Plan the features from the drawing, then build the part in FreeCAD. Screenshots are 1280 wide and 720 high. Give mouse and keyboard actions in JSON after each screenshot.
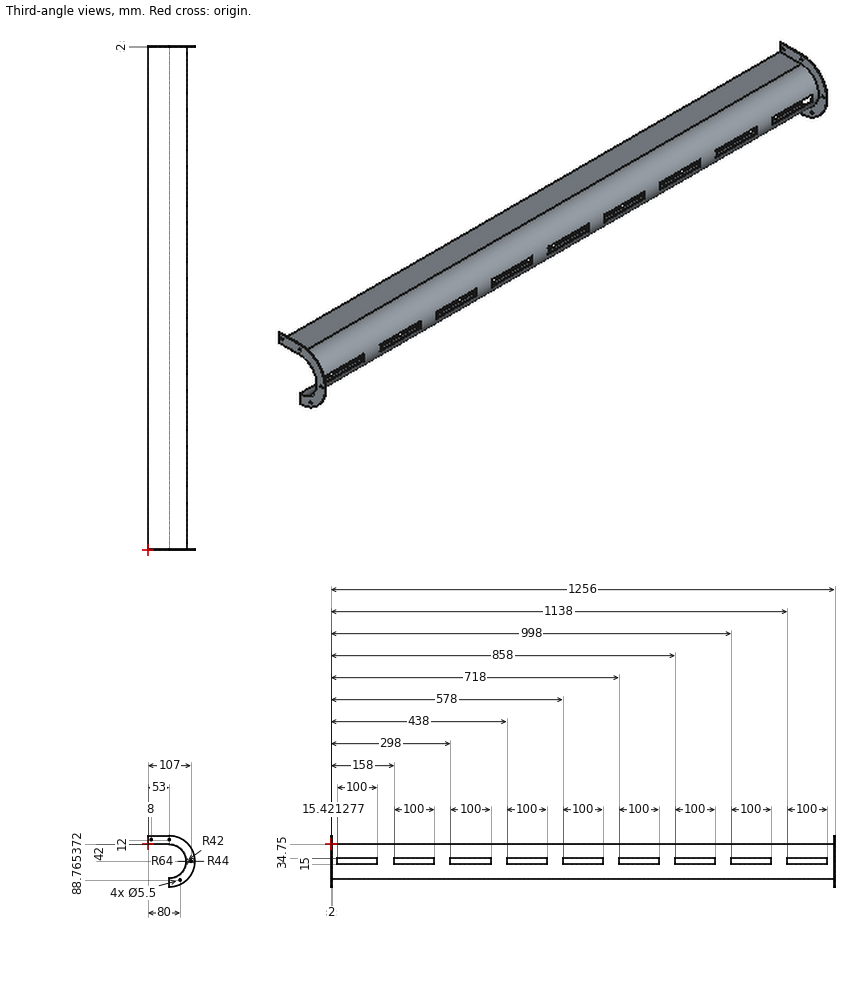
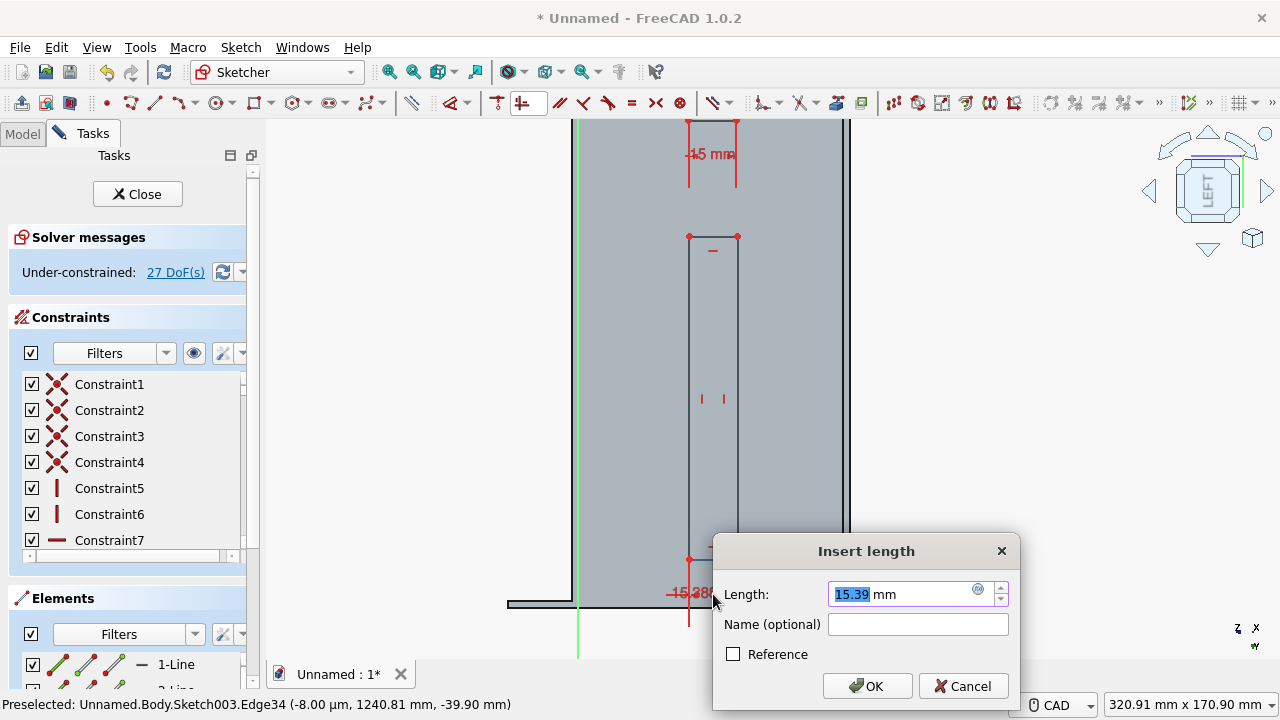
{"action": "type", "text": "15"}
{"action": "key", "text": "Return"}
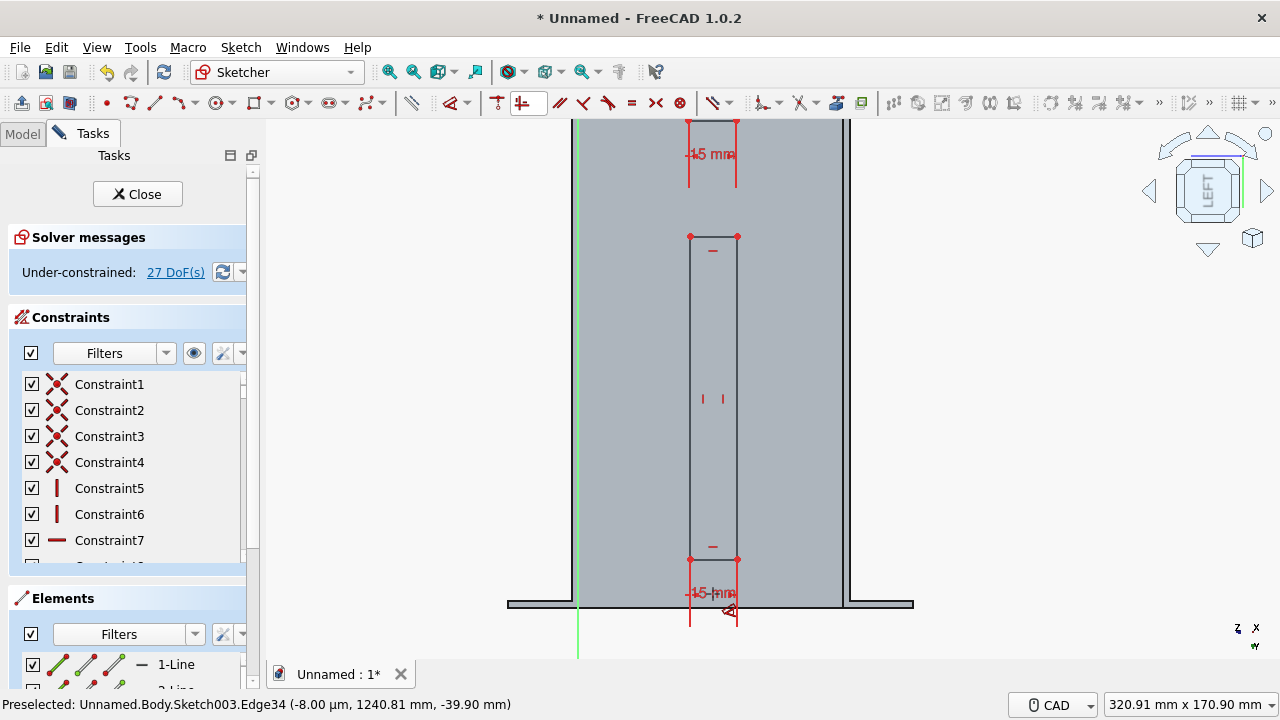
{"action": "scroll", "coordinate": [709, 568], "scroll_direction": "down", "scroll_amount": 12}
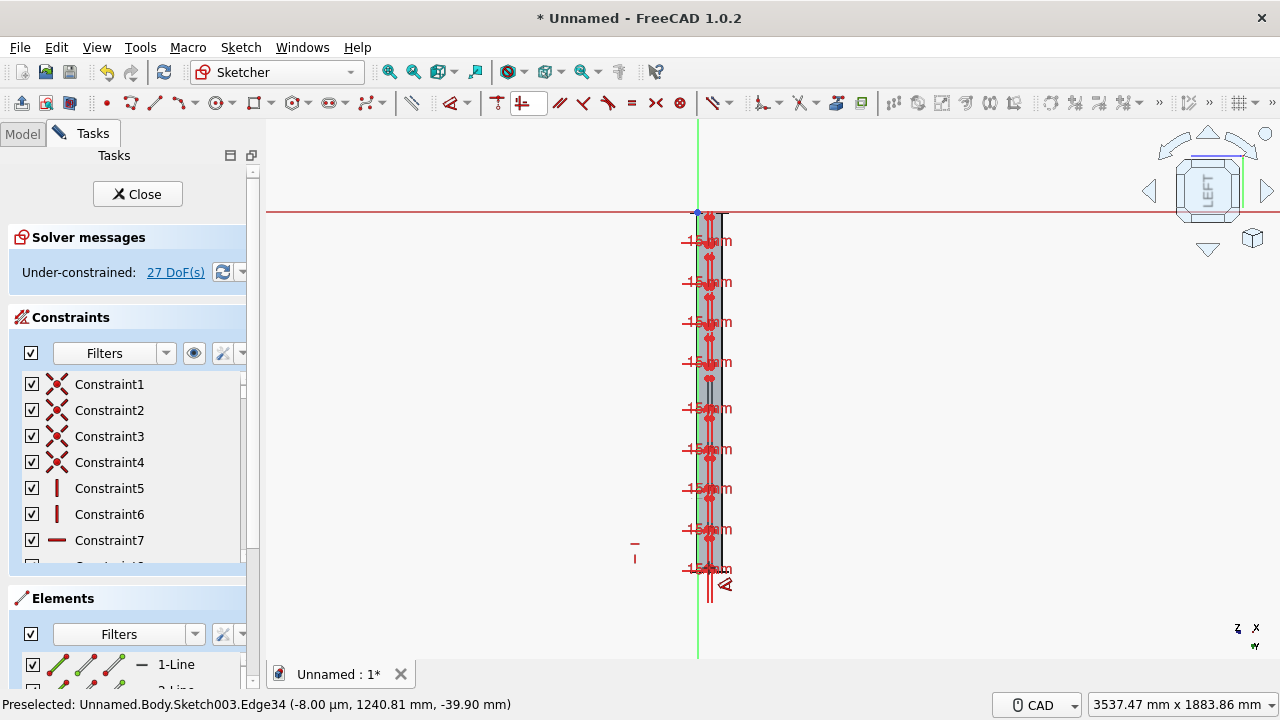
{"action": "scroll", "coordinate": [708, 226], "scroll_direction": "up", "scroll_amount": 6}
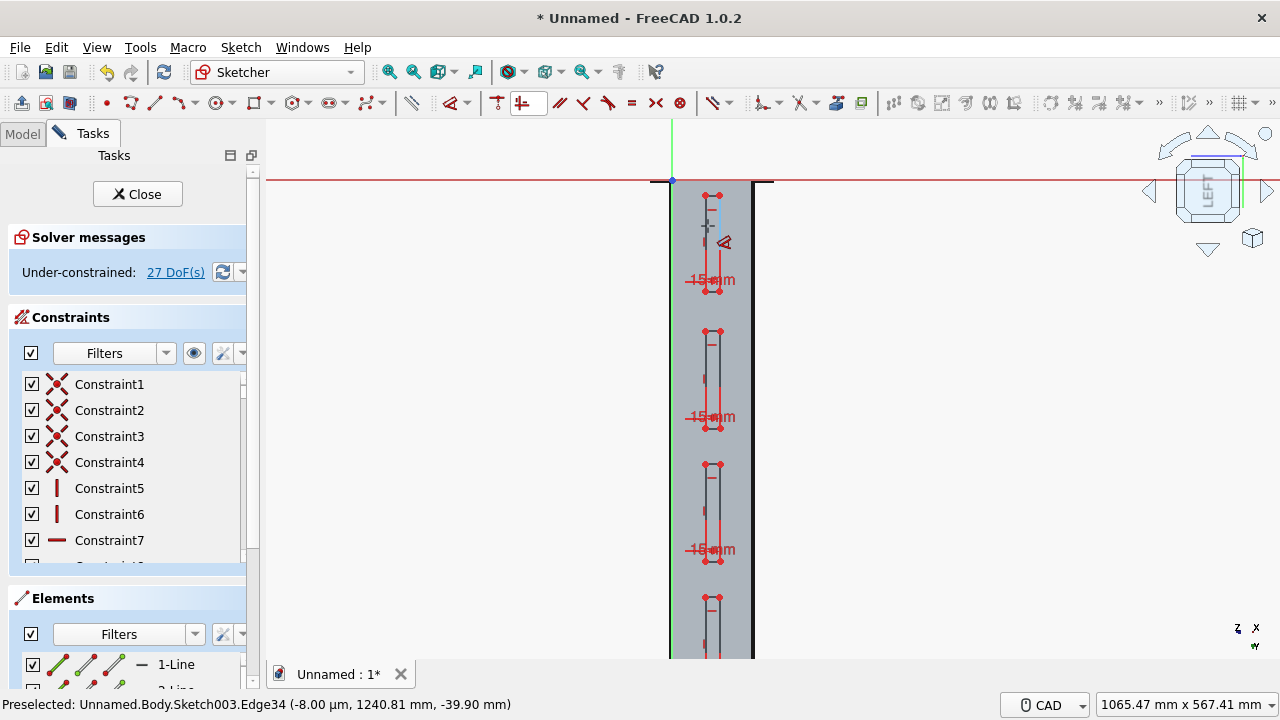
{"action": "left_click", "coordinate": [706, 225]}
{"action": "left_click", "coordinate": [740, 244]}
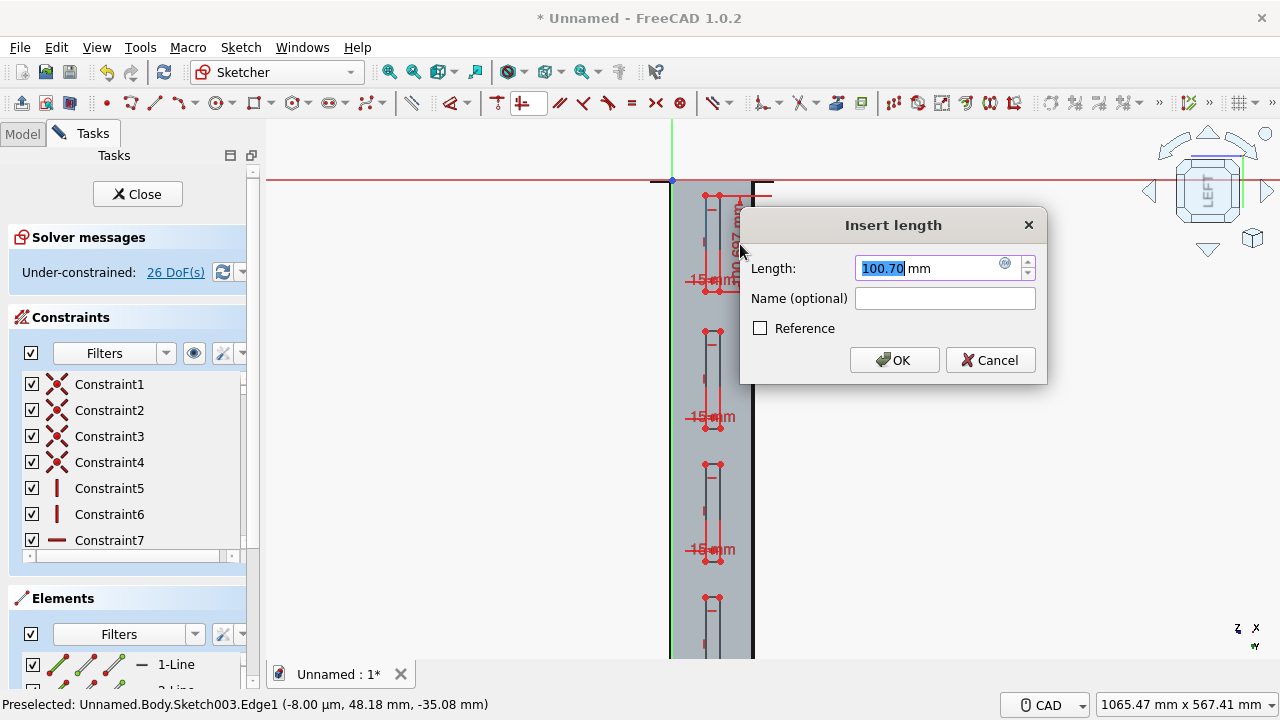
{"action": "type", "text": "100"}
{"action": "key", "text": "Return"}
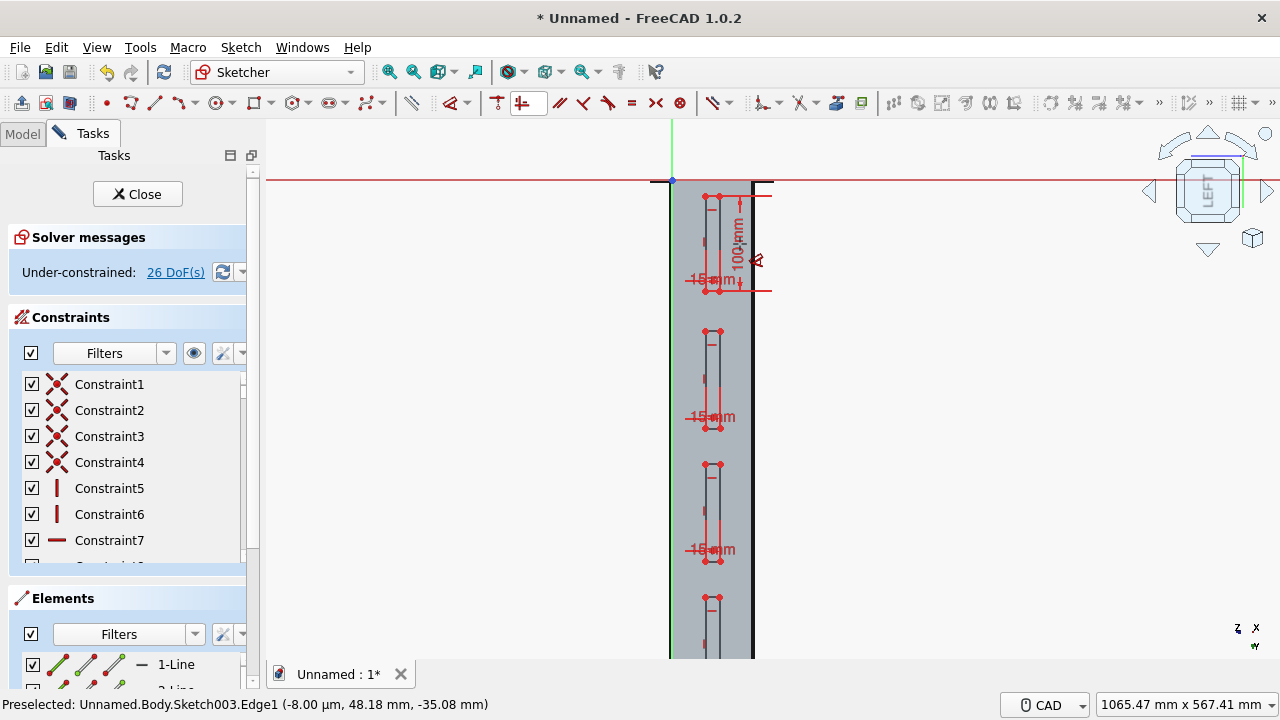
{"action": "left_click", "coordinate": [706, 361]}
{"action": "left_click", "coordinate": [740, 380]}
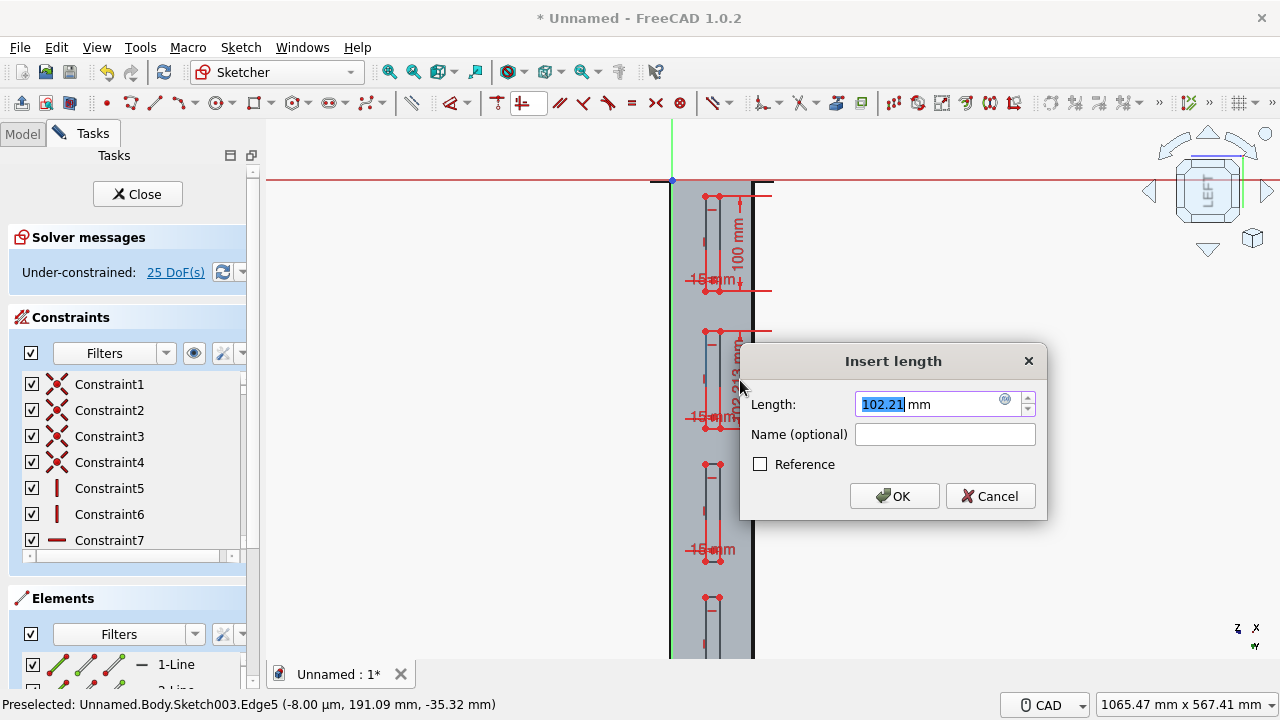
{"action": "type", "text": "100"}
{"action": "key", "text": "Return"}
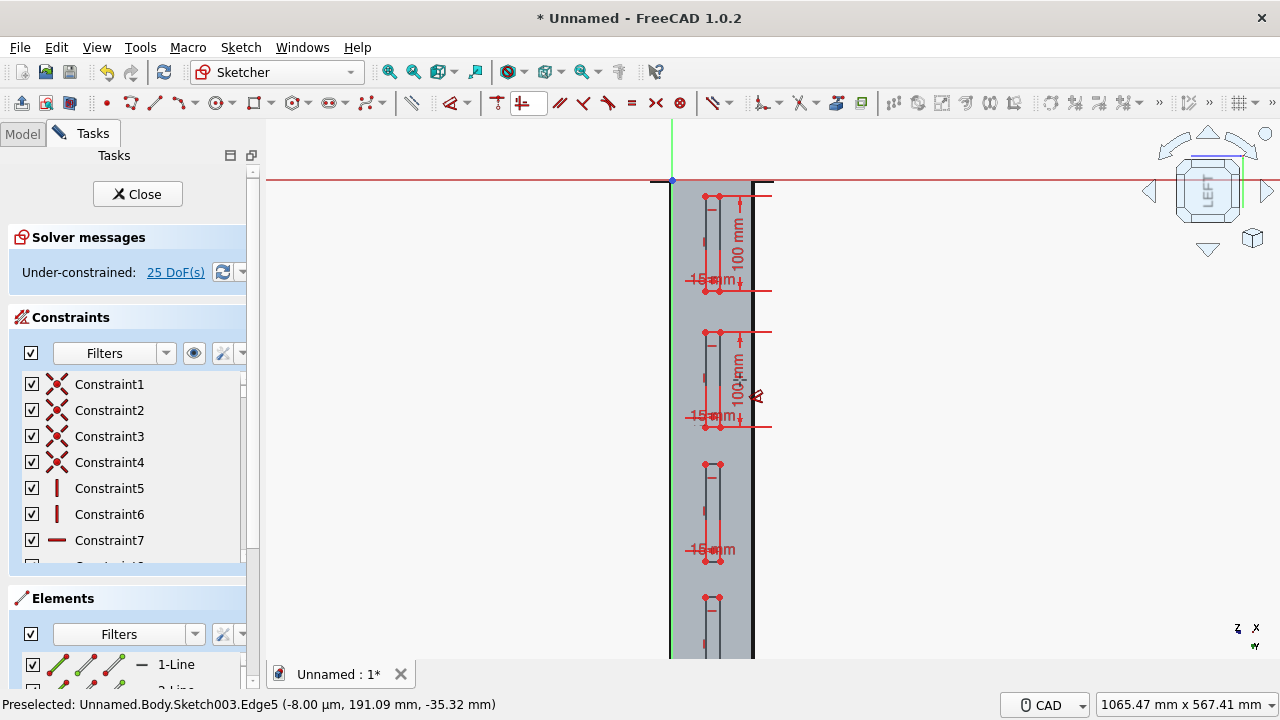
{"action": "scroll", "coordinate": [708, 225], "scroll_direction": "down", "scroll_amount": 6}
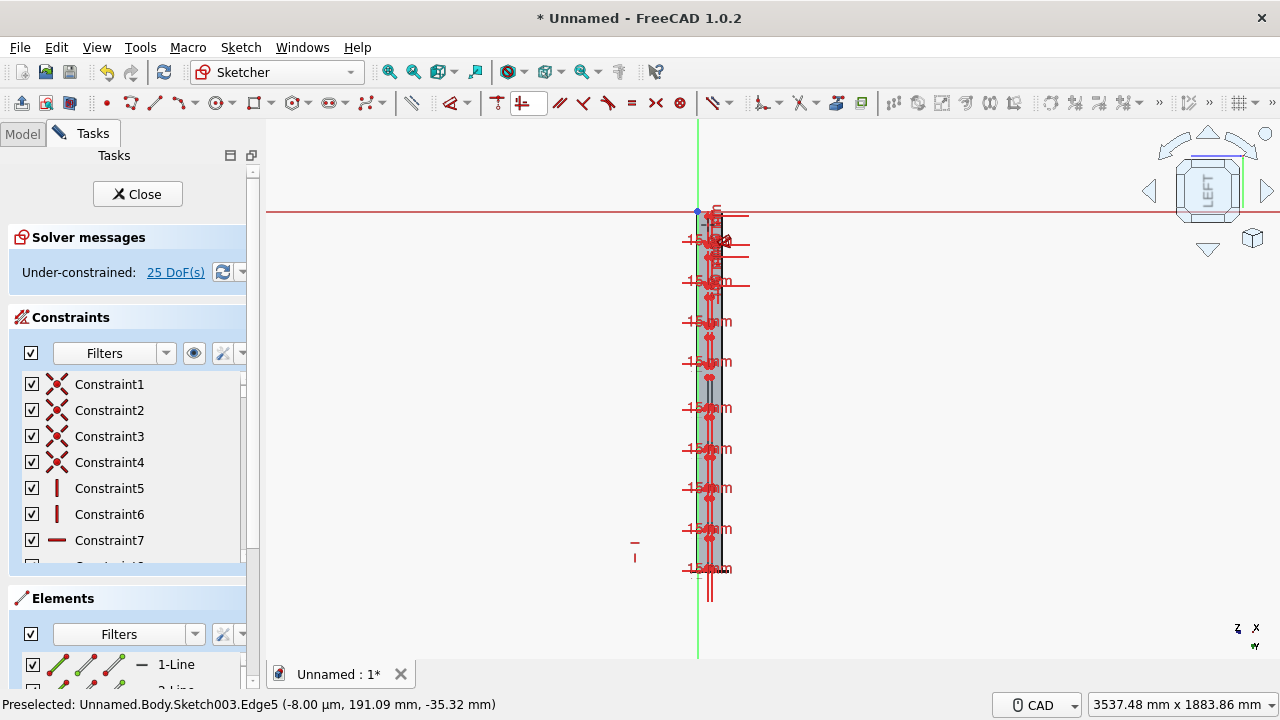
{"action": "scroll", "coordinate": [708, 507], "scroll_direction": "up", "scroll_amount": 6}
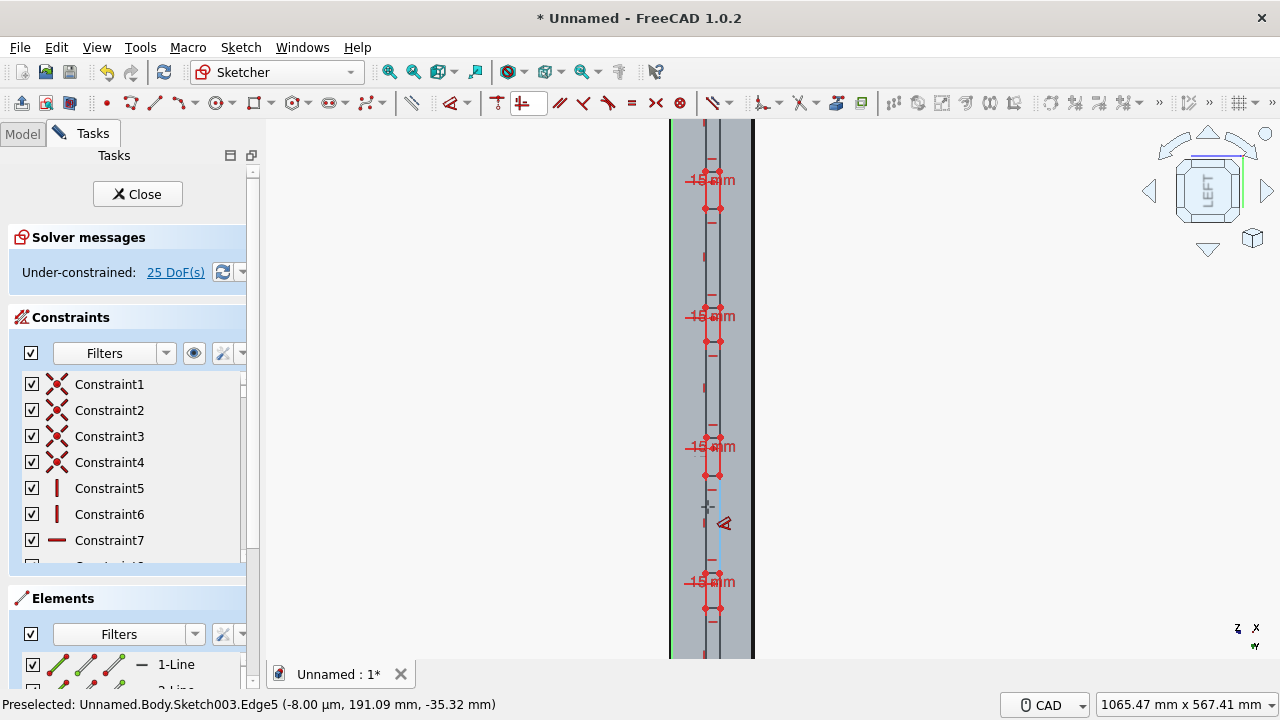
{"action": "left_click", "coordinate": [706, 505]}
{"action": "left_click", "coordinate": [740, 524]}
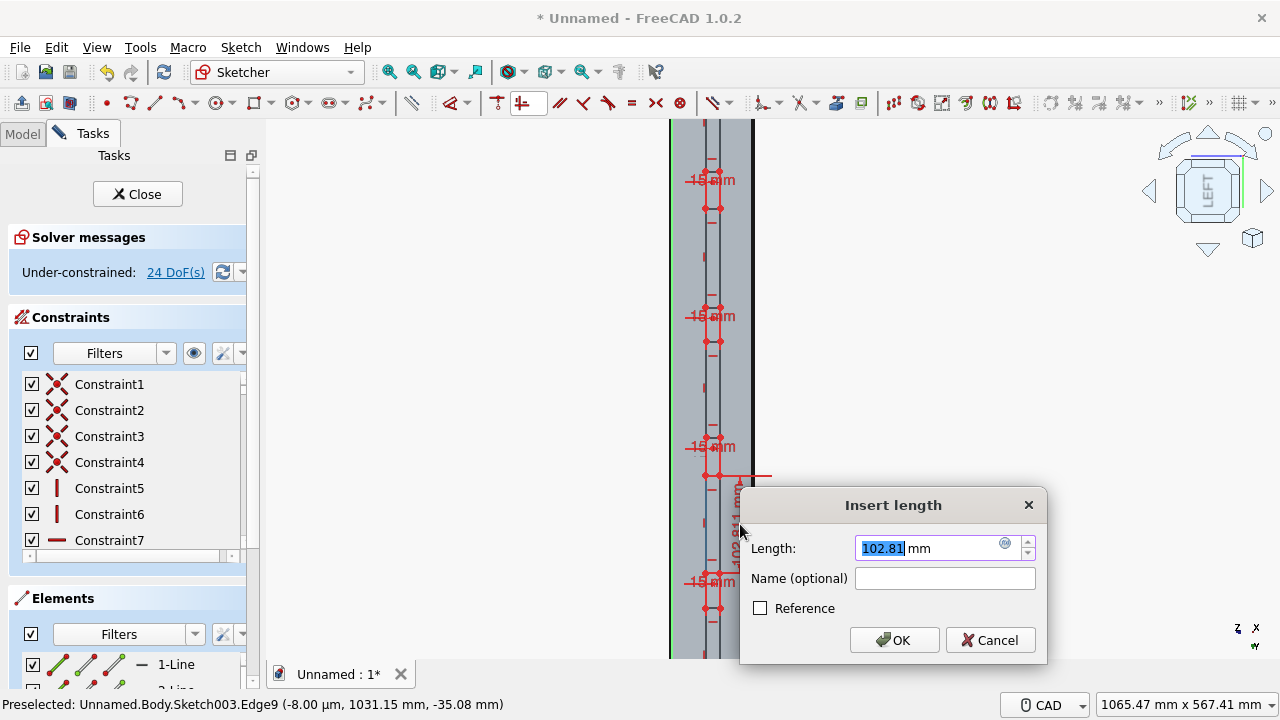
{"action": "type", "text": "100"}
{"action": "key", "text": "Return"}